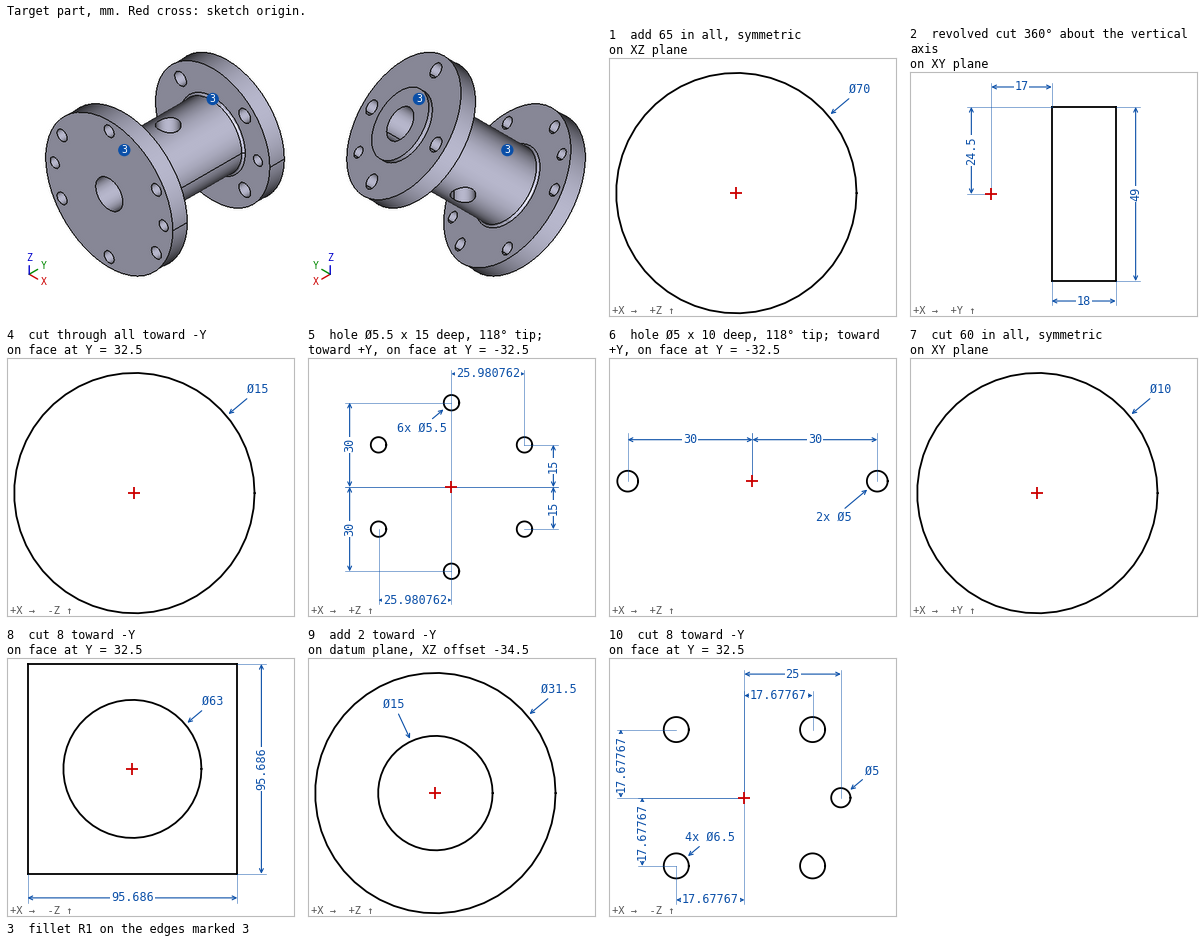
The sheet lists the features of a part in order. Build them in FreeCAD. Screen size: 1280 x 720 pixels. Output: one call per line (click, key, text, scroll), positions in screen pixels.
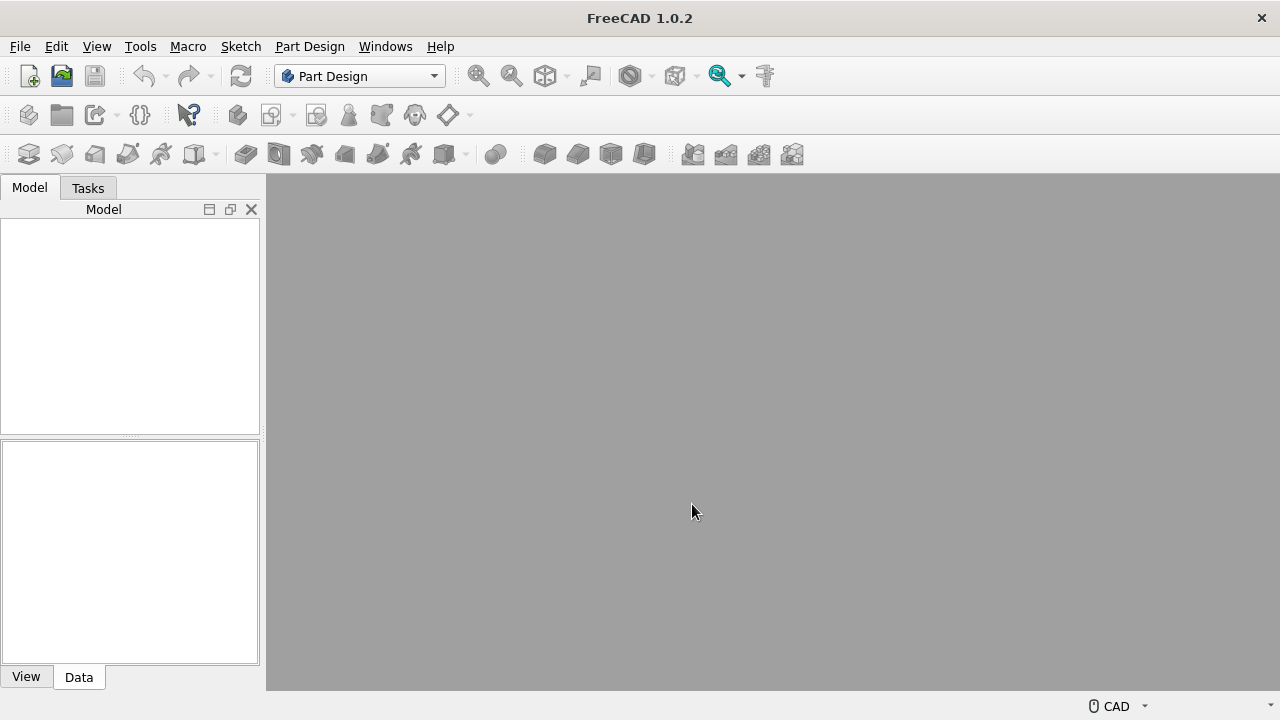
click(29, 76)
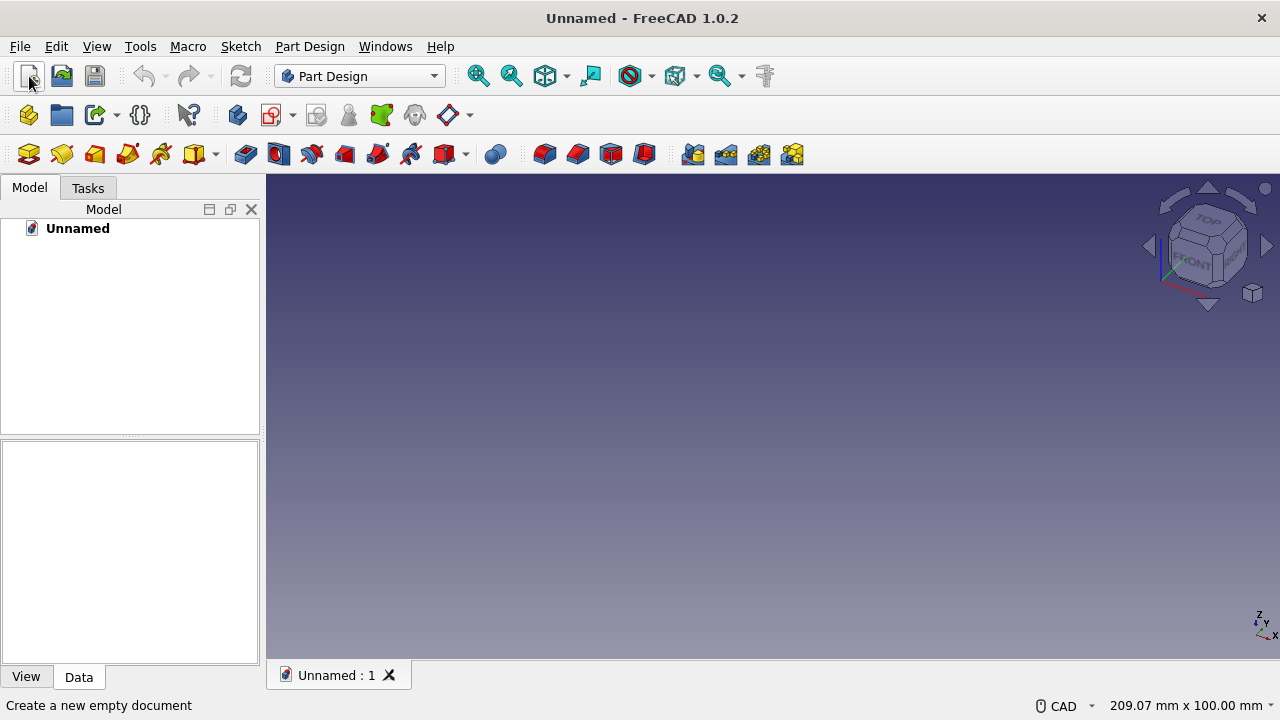
click(270, 116)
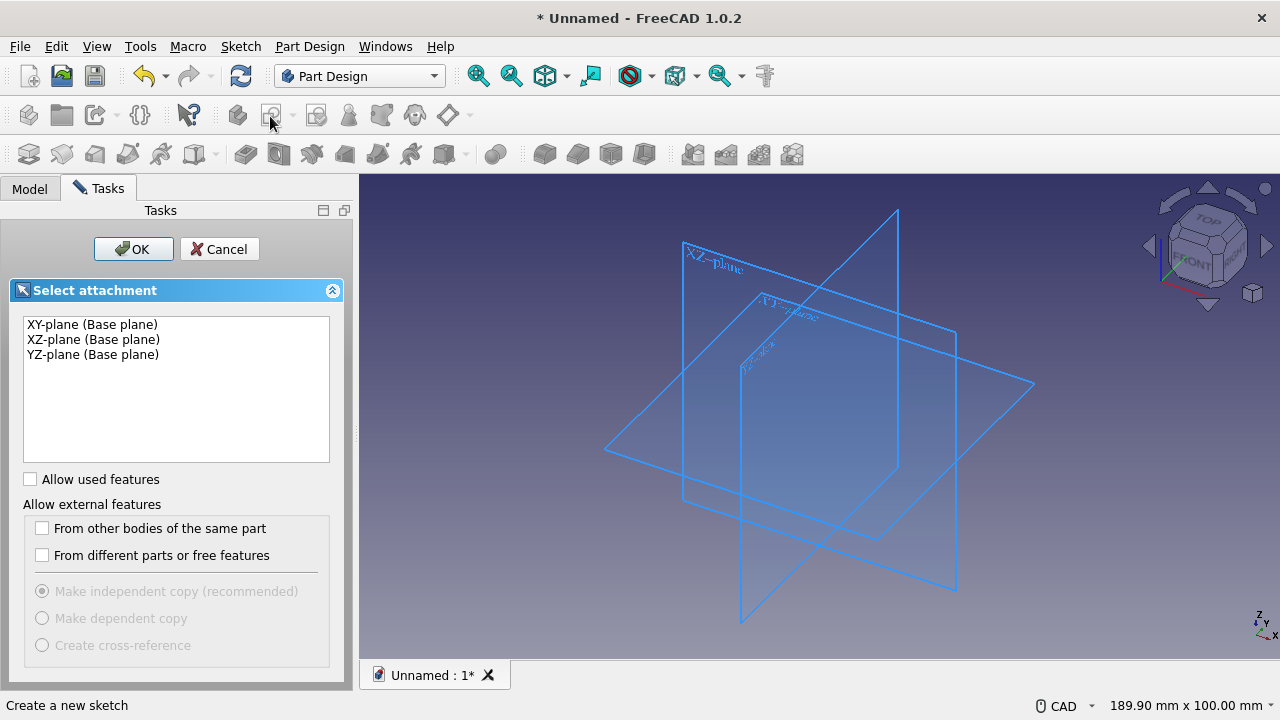
click(84, 340)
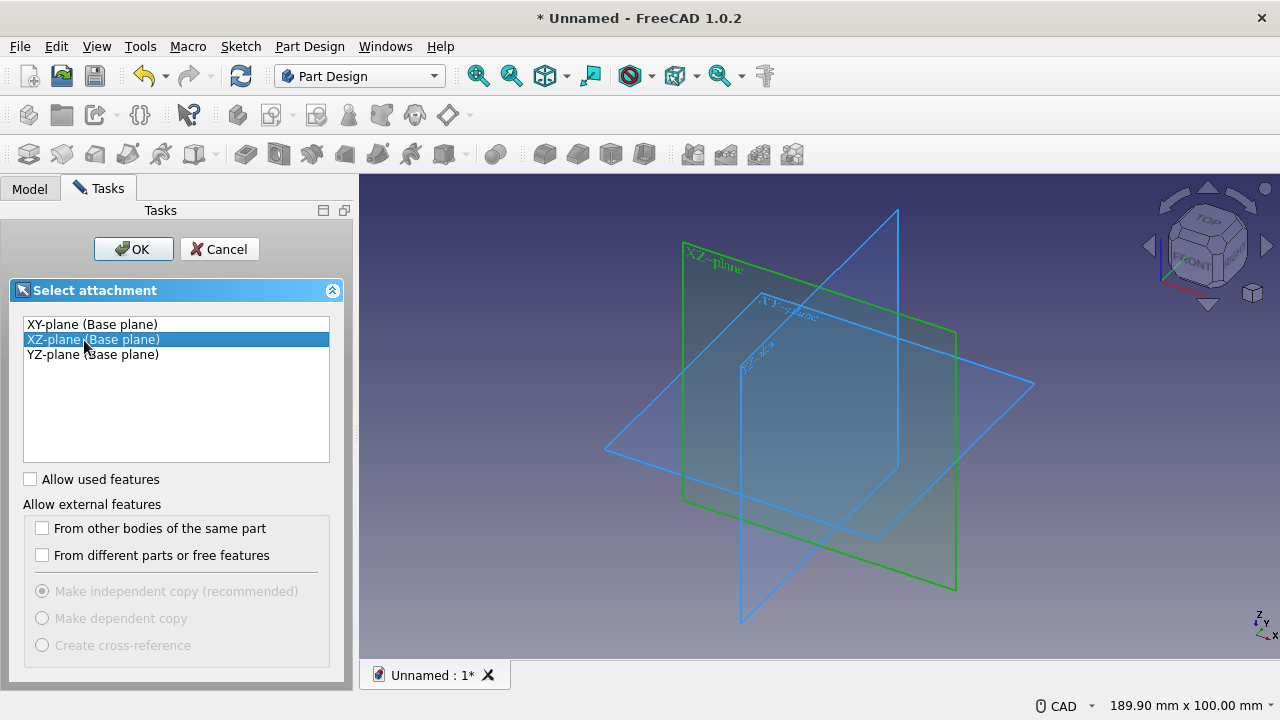
click(134, 249)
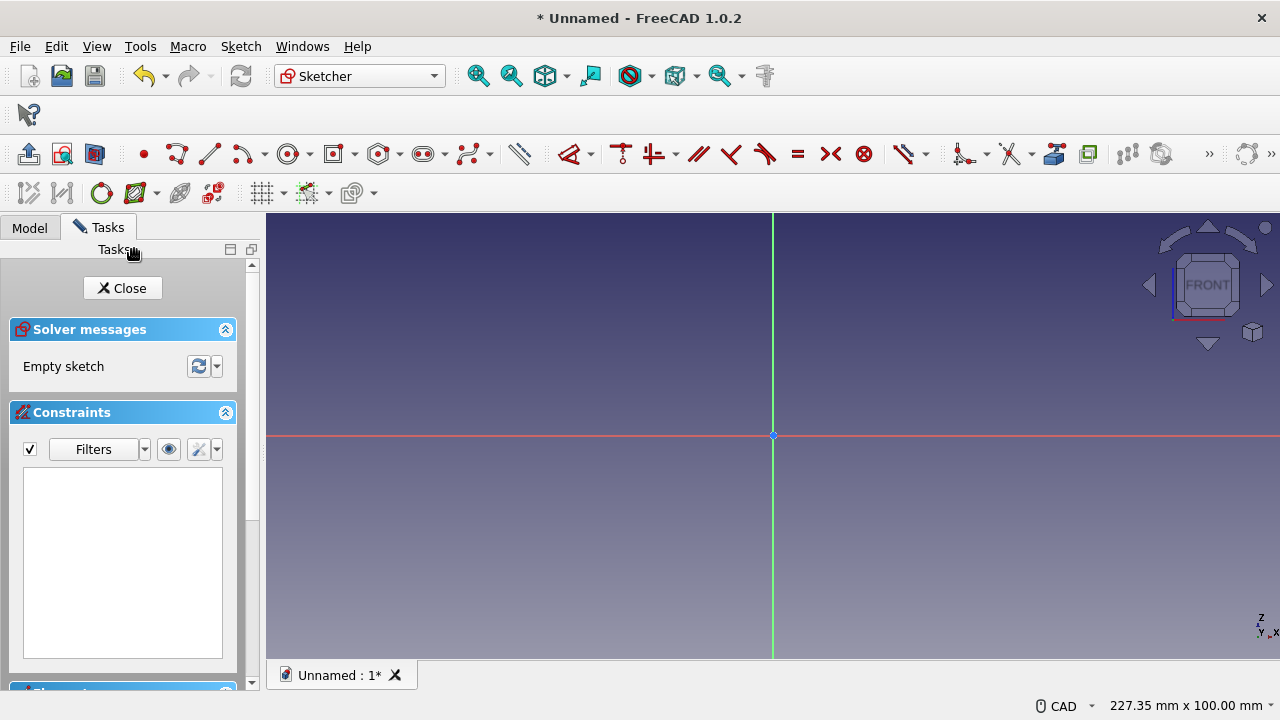
click(288, 154)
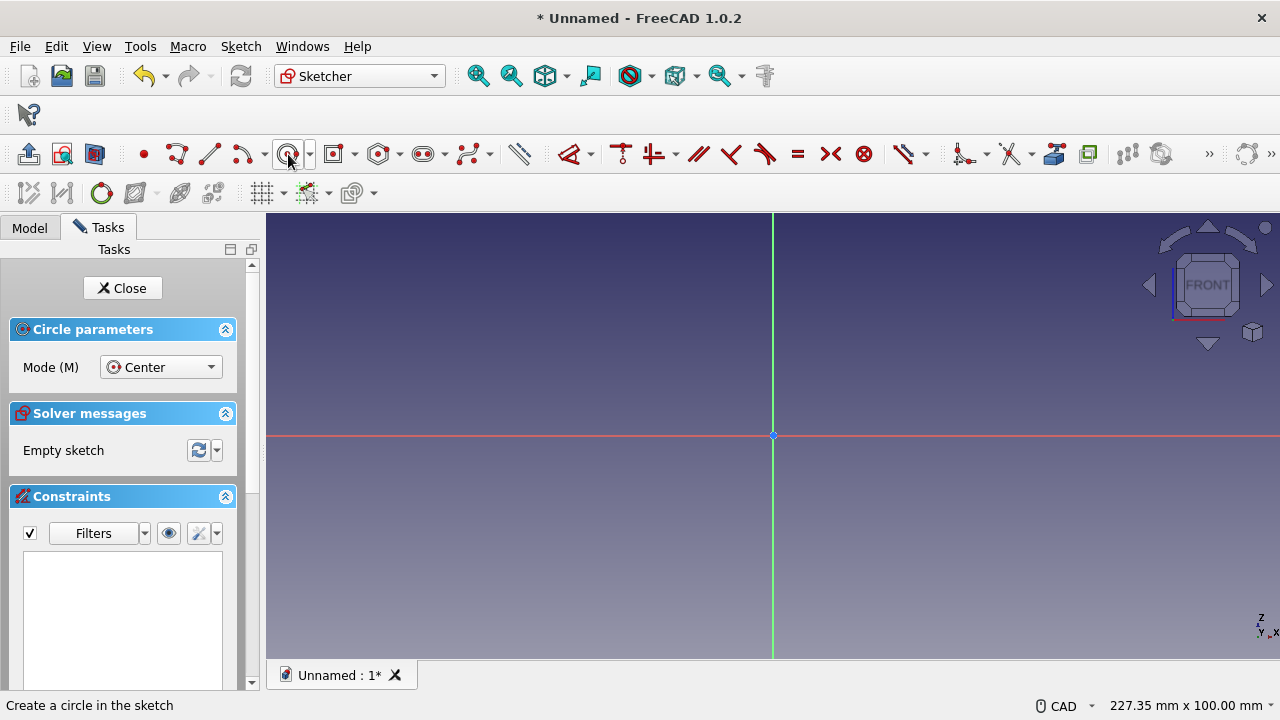
click(773, 436)
move(883, 326)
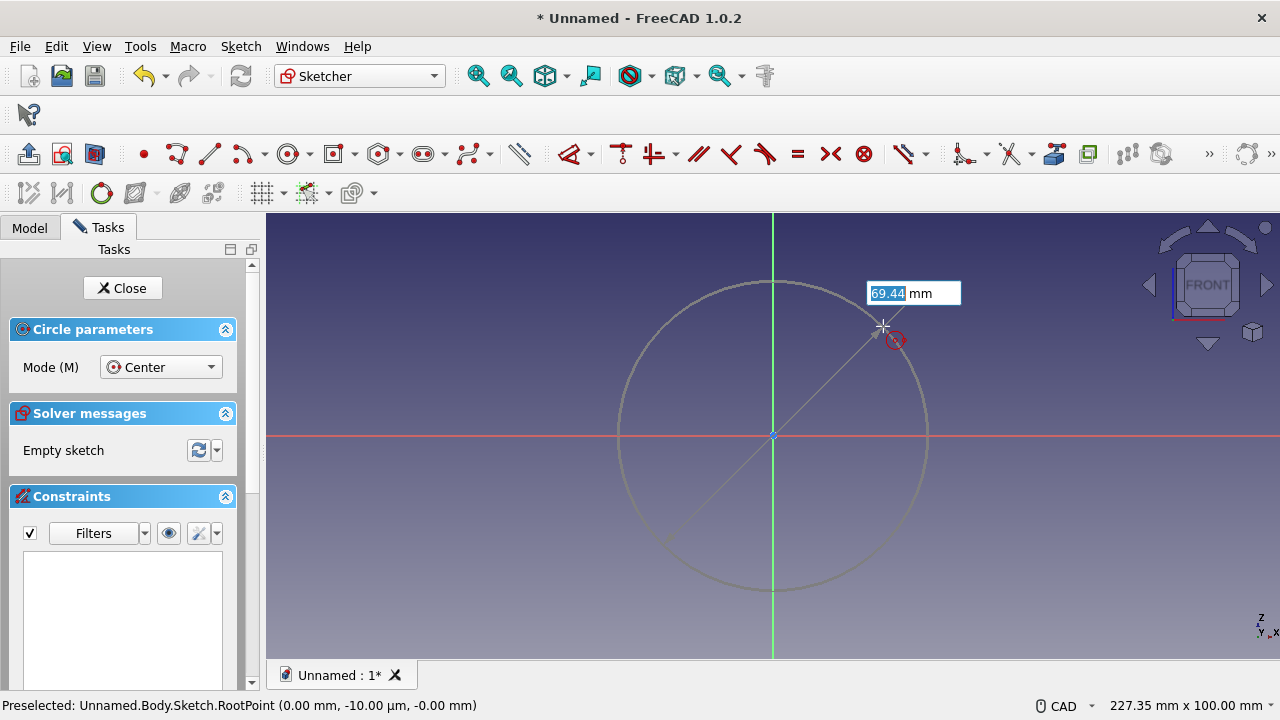
text(70)
key(Return)
key(Escape)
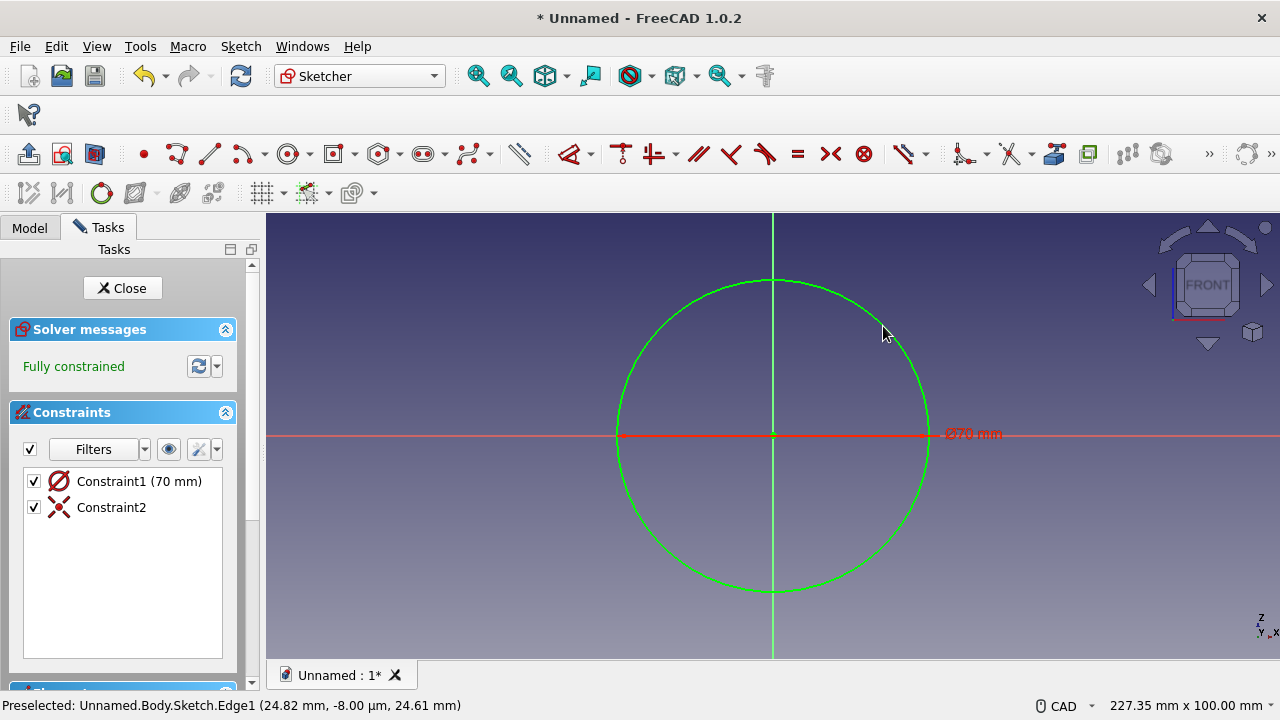
click(123, 288)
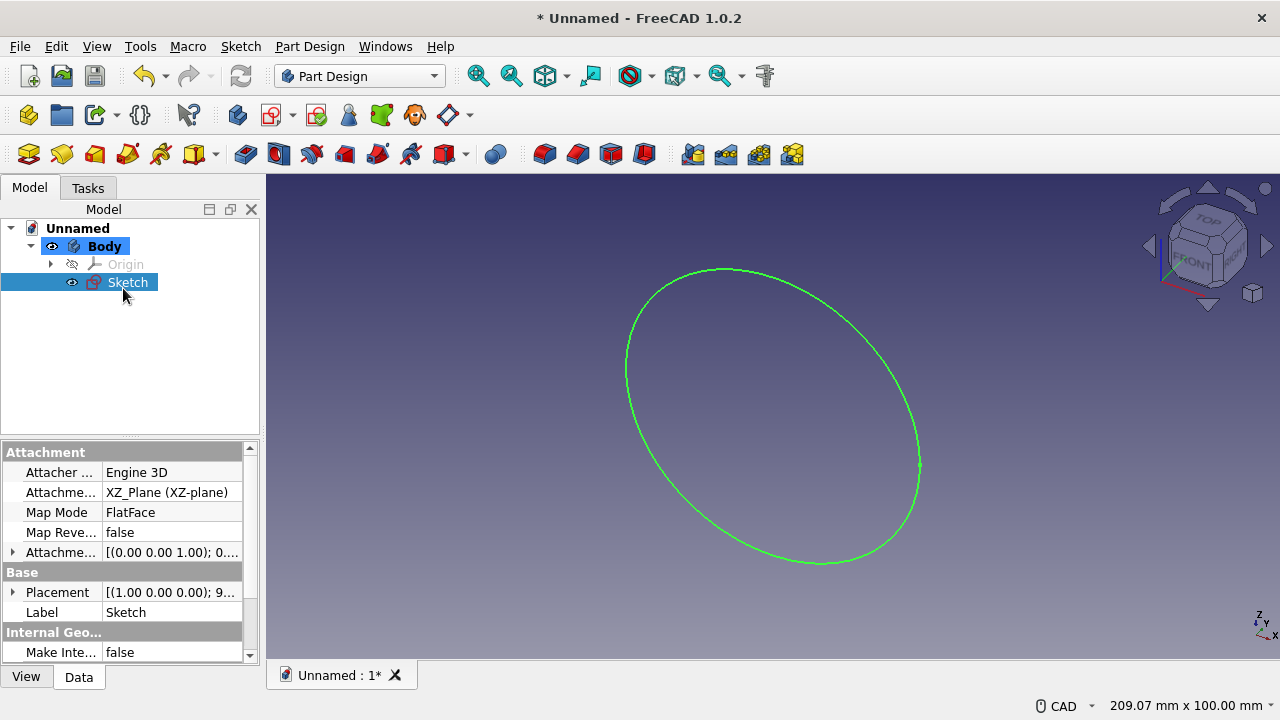
click(29, 154)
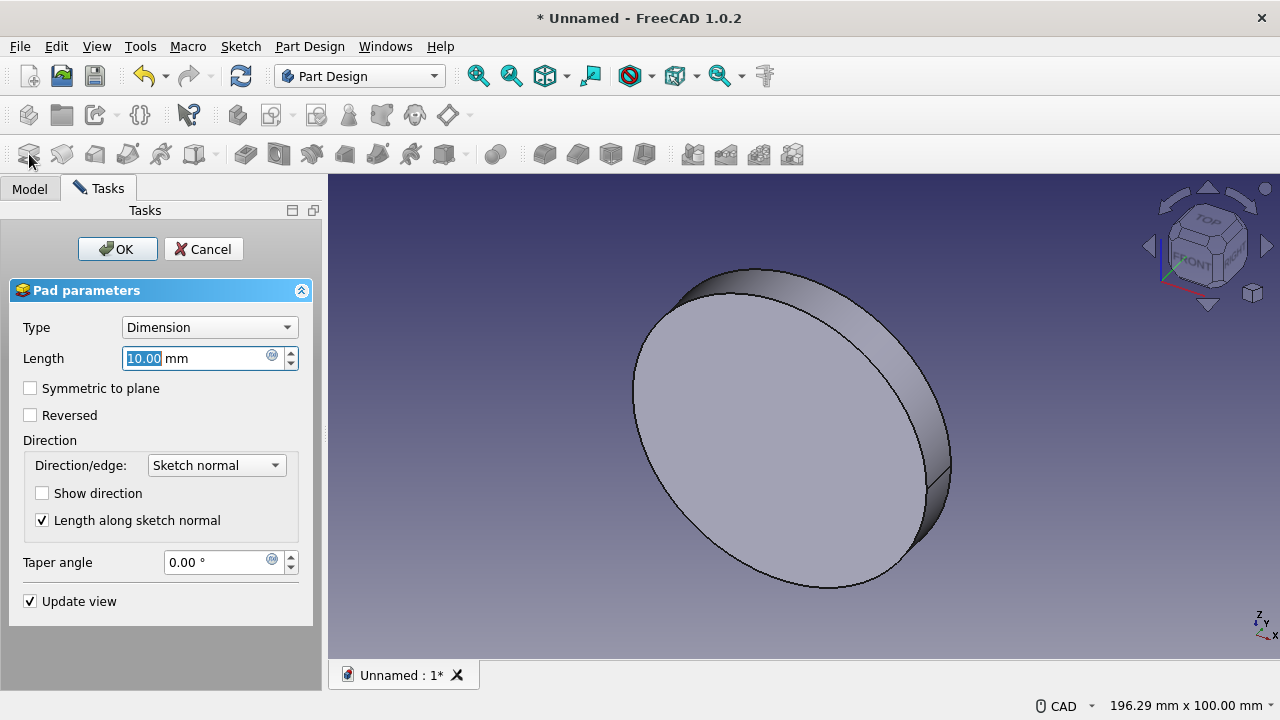
text(65)
key(Tab)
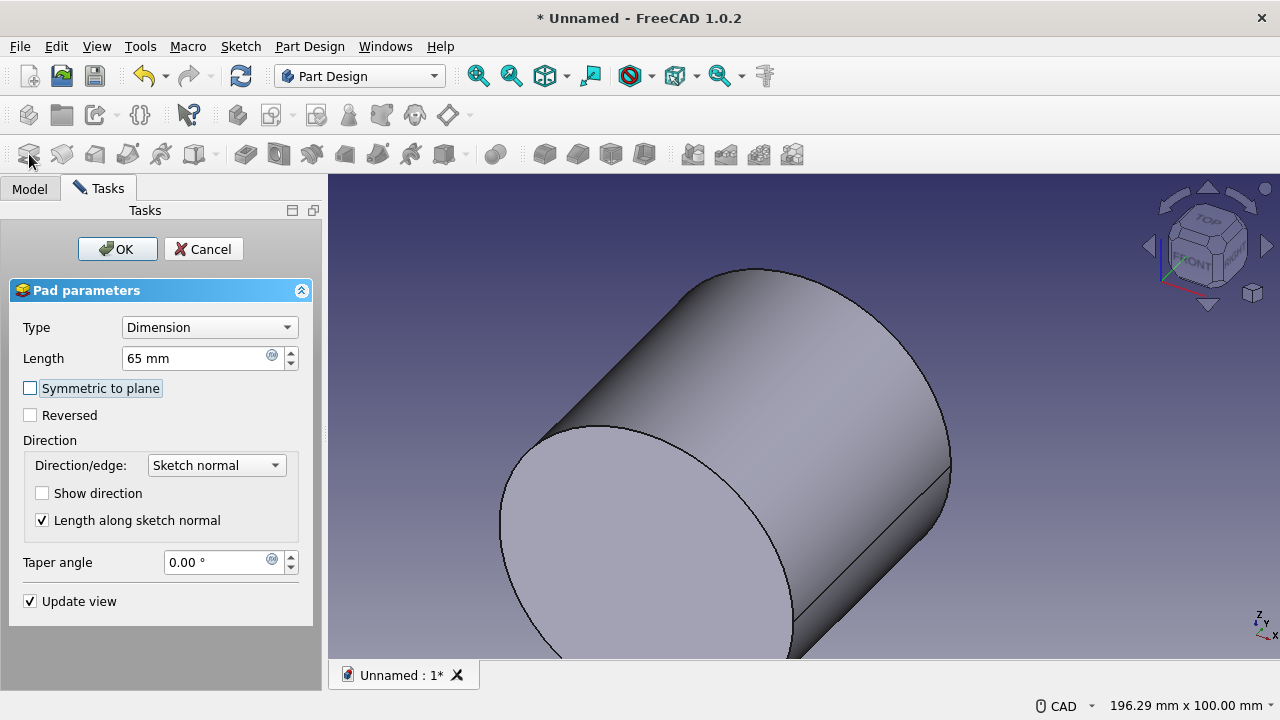
click(31, 388)